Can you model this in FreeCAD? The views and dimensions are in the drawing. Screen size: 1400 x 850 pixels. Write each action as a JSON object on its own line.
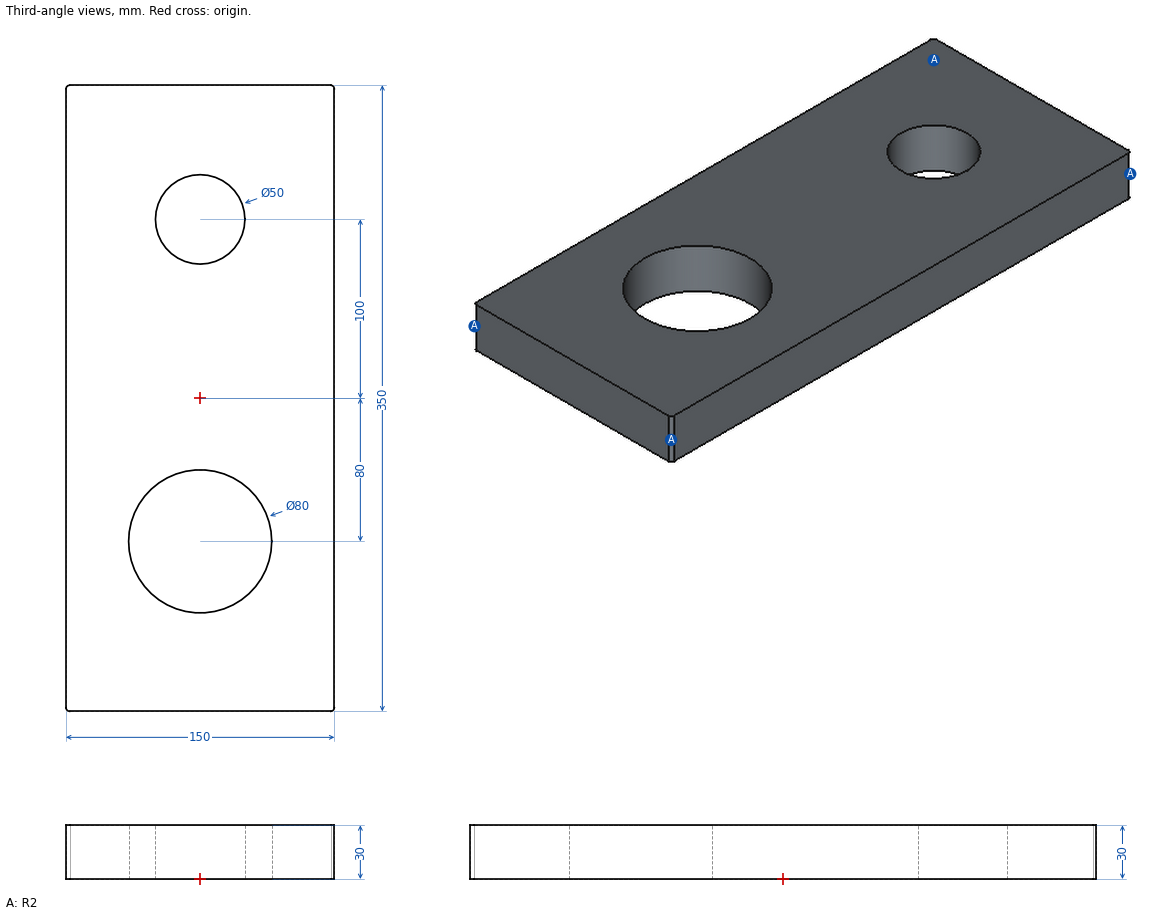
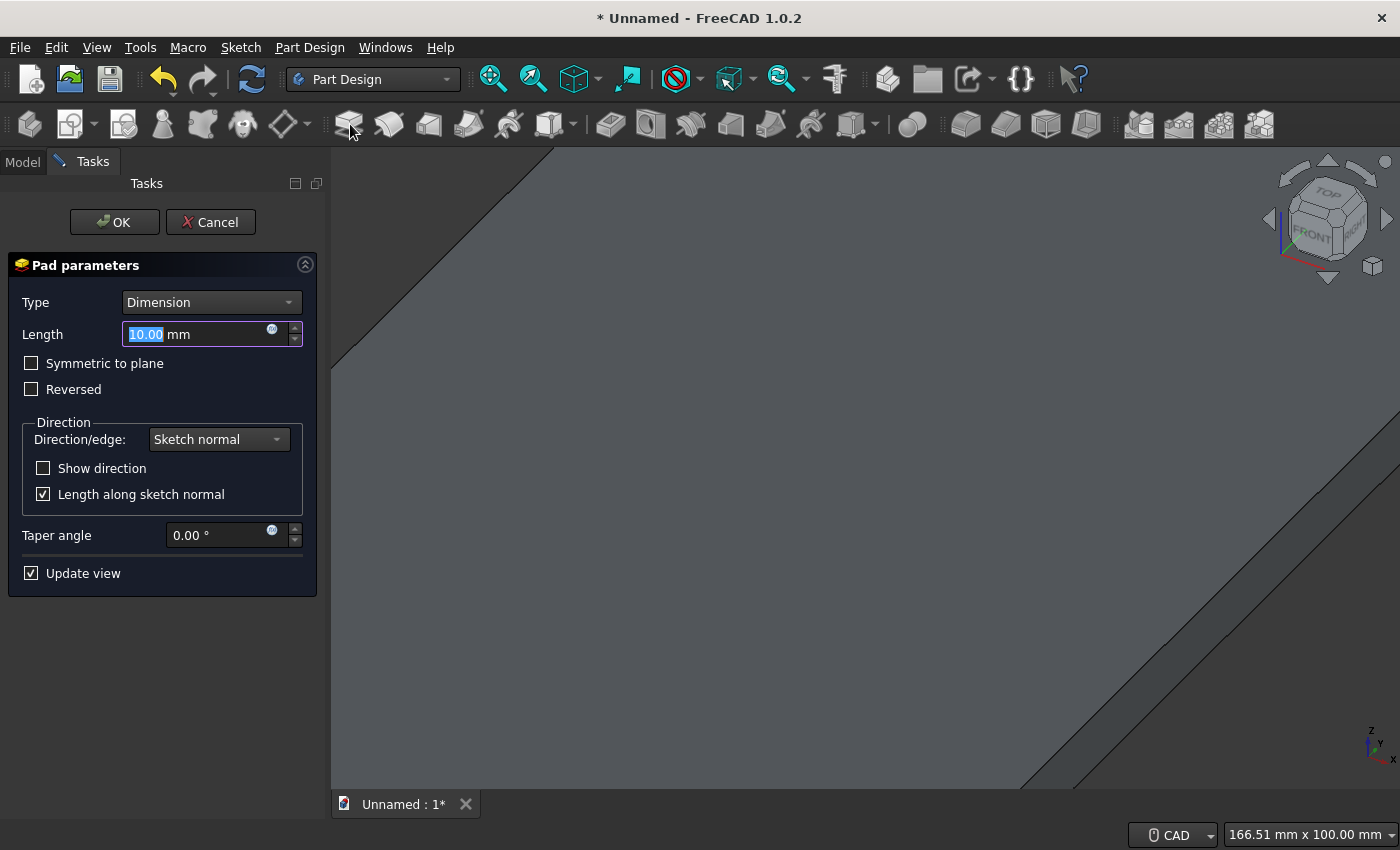
{"action": "type", "text": "30"}
{"action": "key", "text": "Tab"}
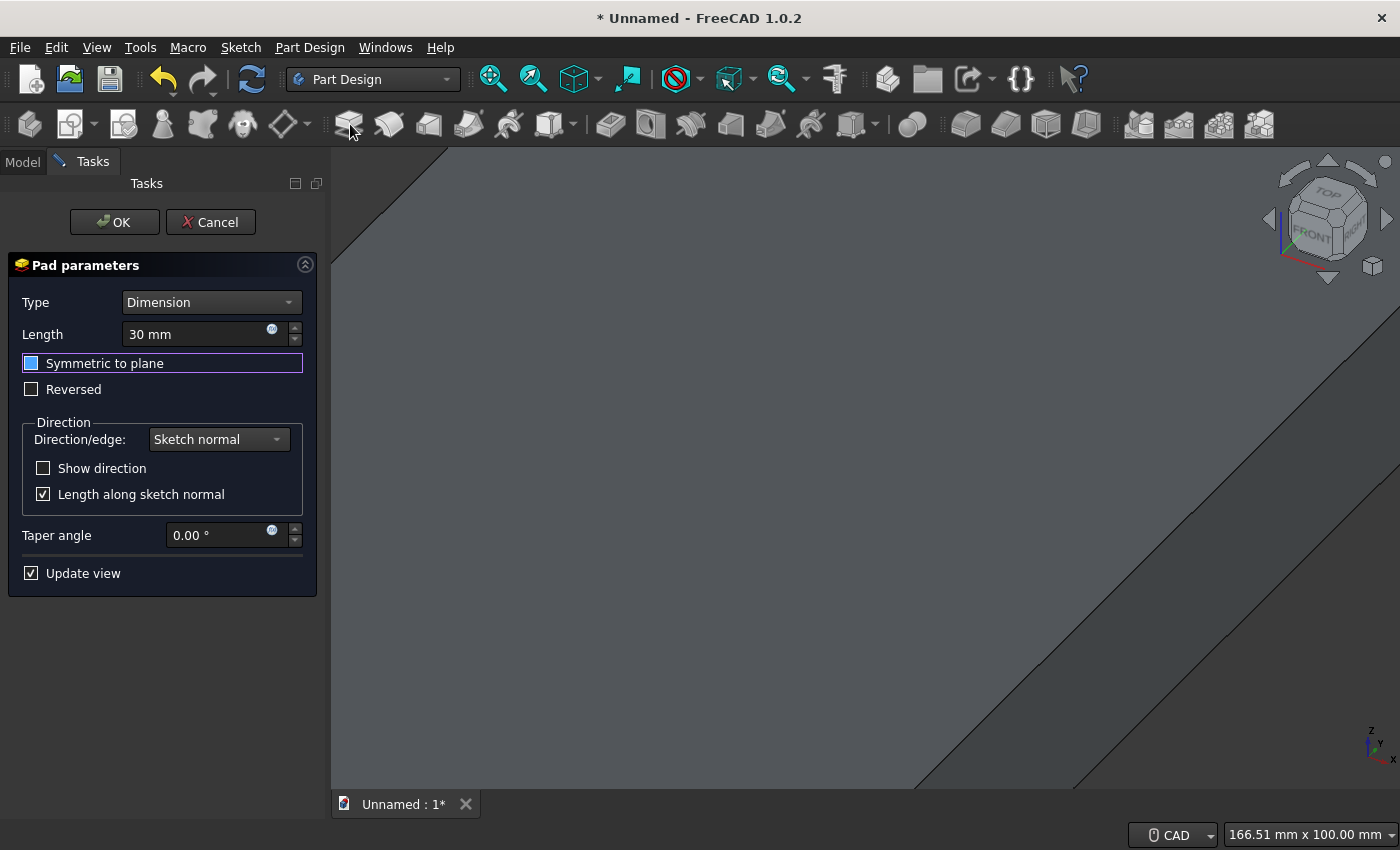
{"action": "left_click", "coordinate": [115, 222]}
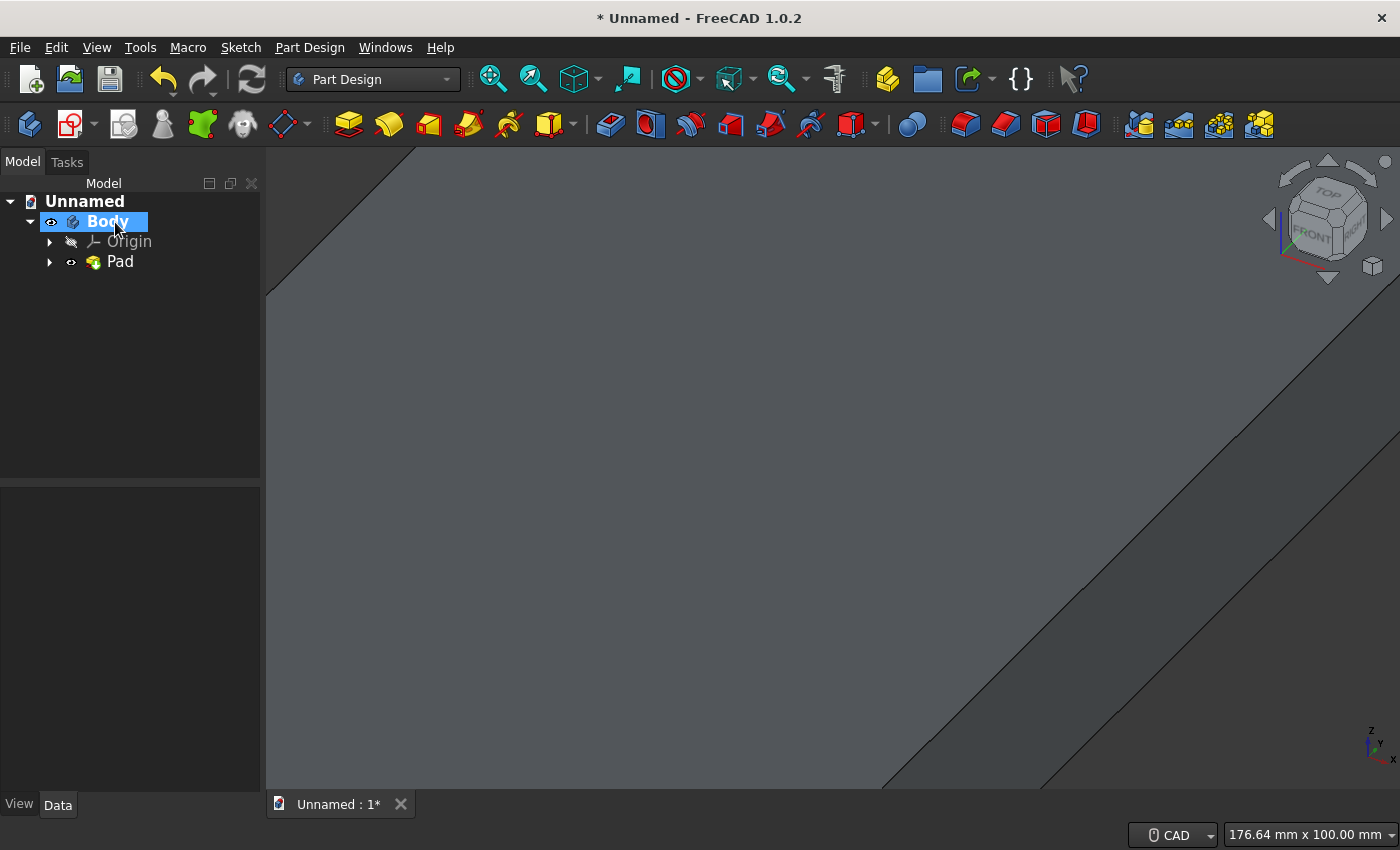
{"action": "left_click", "coordinate": [494, 80]}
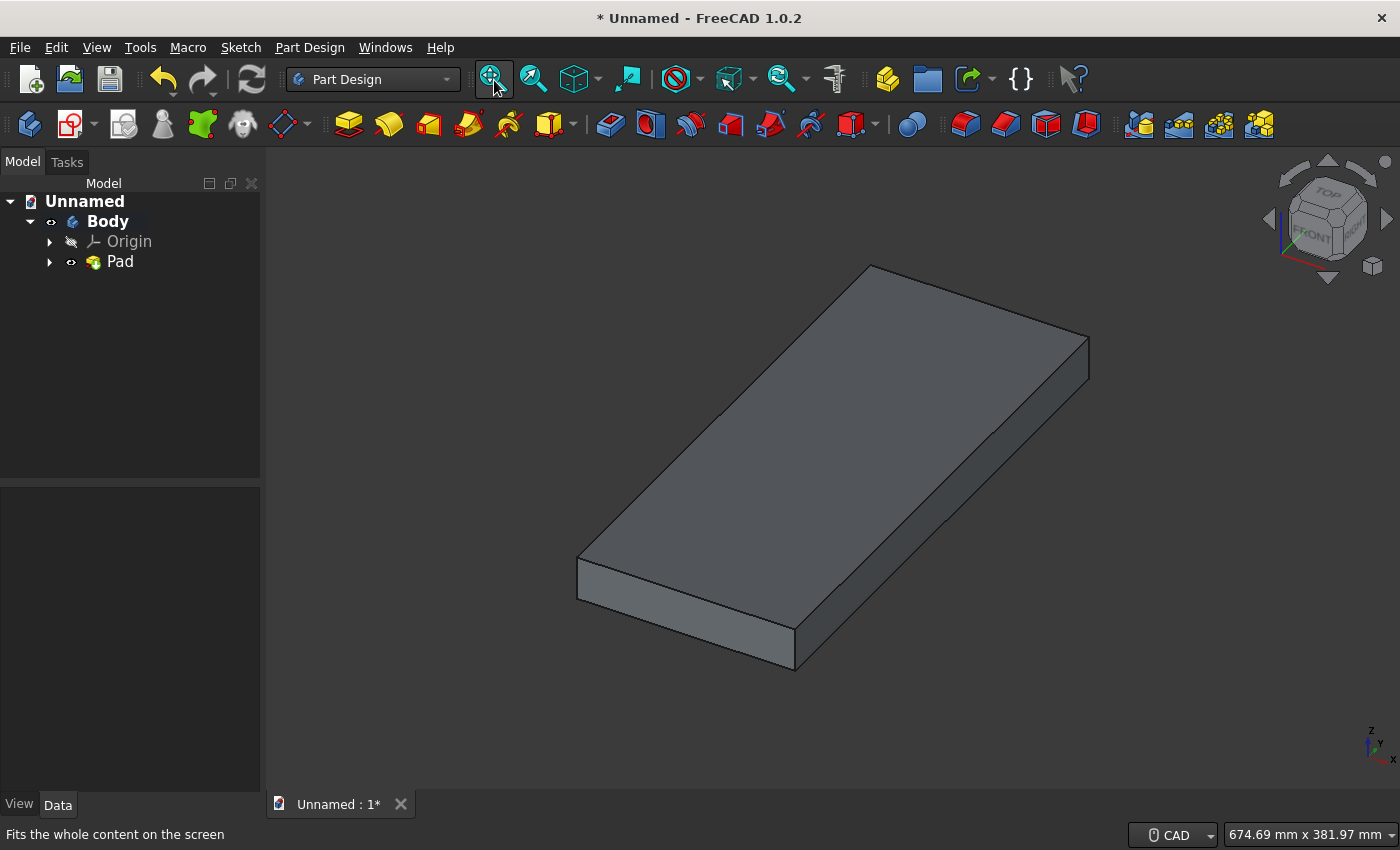
{"action": "left_click", "coordinate": [917, 363]}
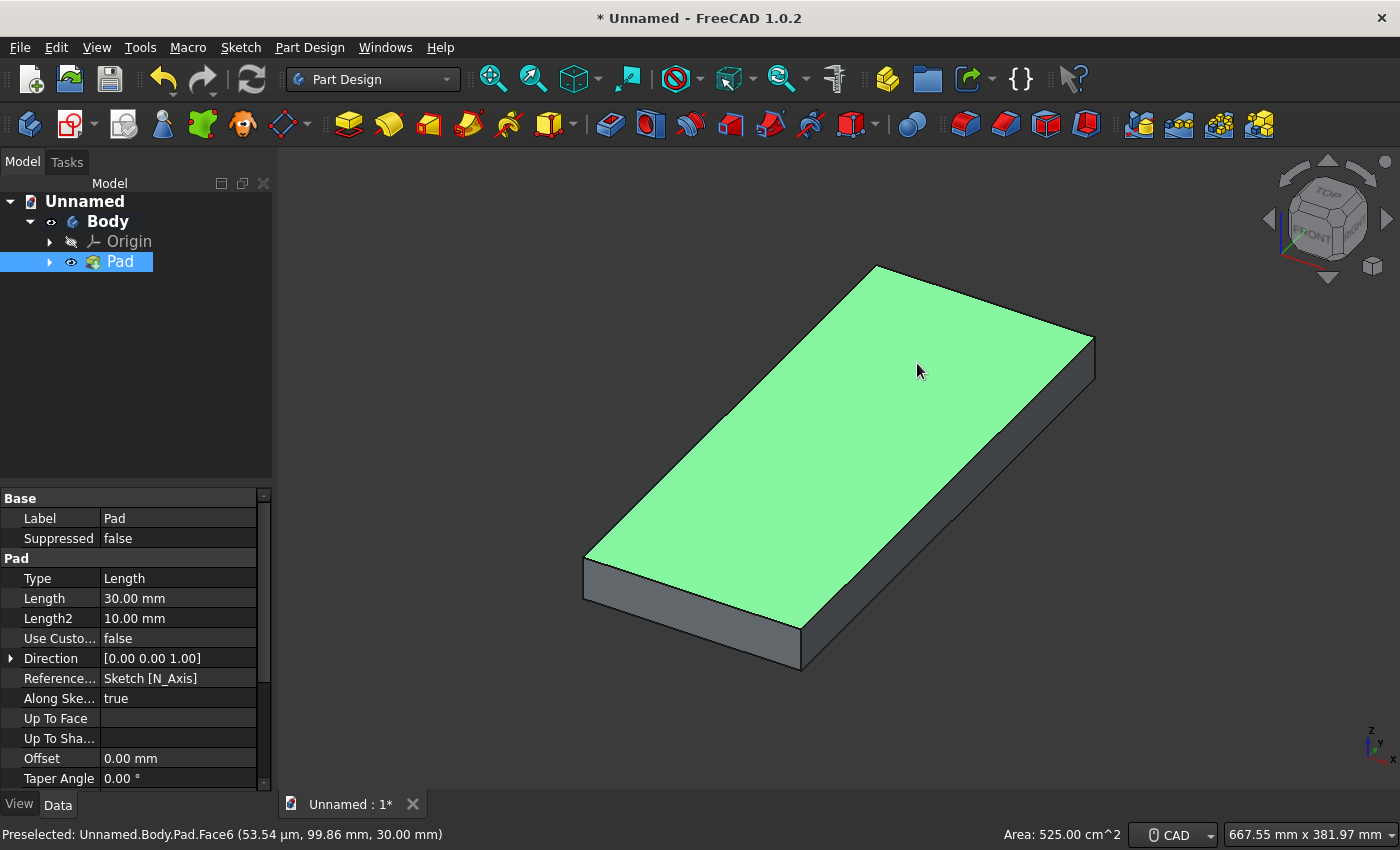
{"action": "left_click", "coordinate": [70, 124]}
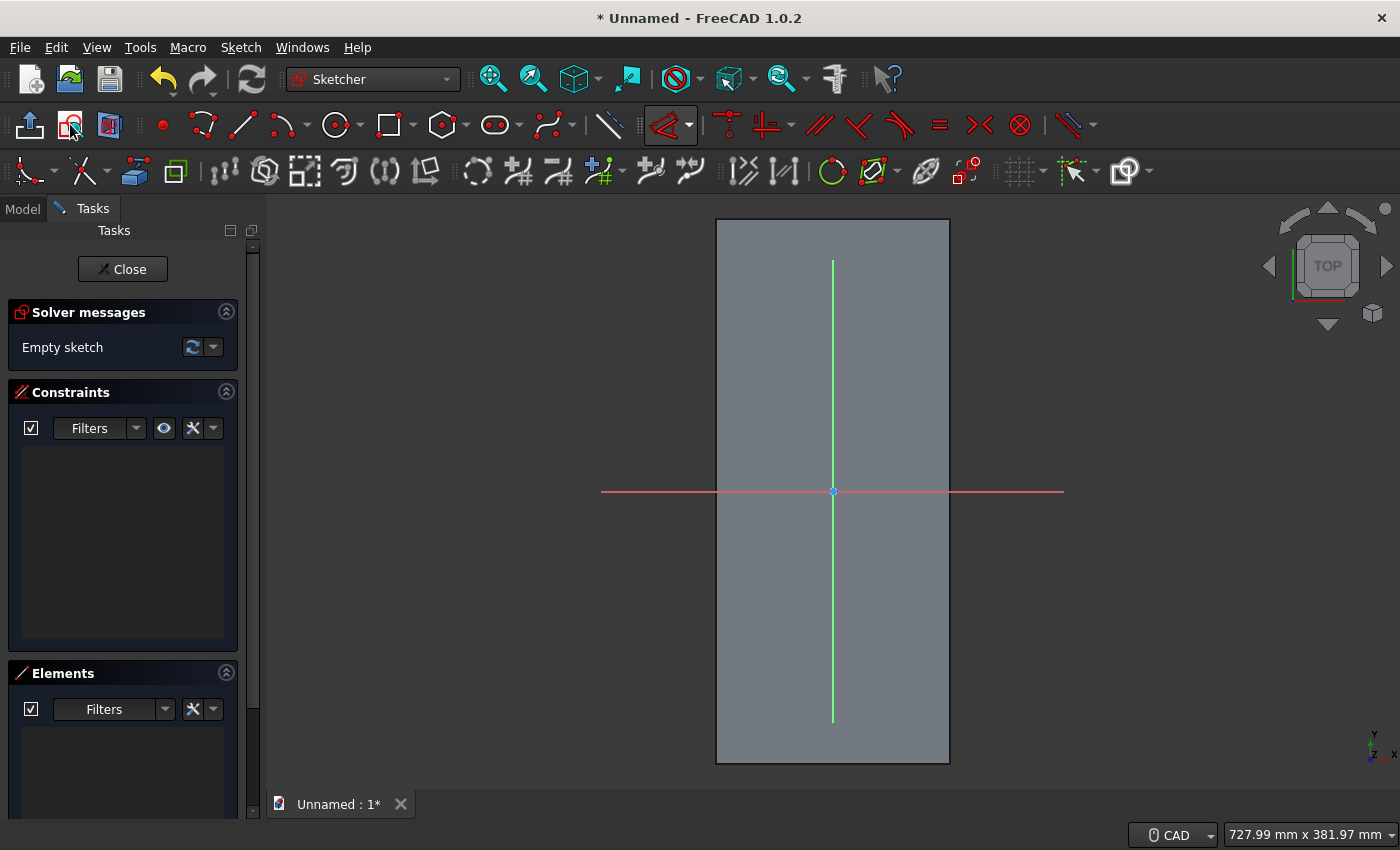
{"action": "left_click", "coordinate": [336, 126]}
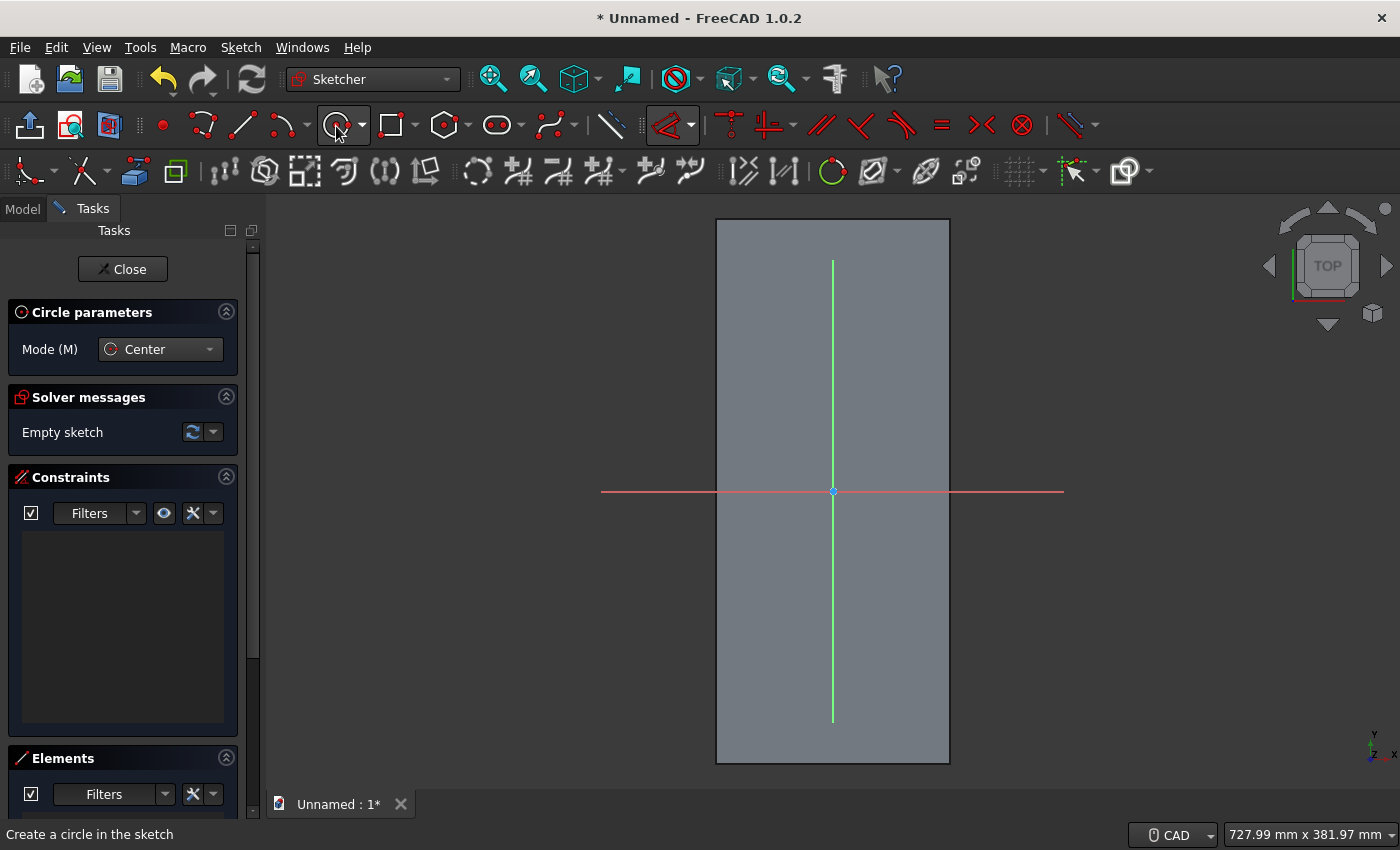
{"action": "left_click", "coordinate": [833, 336]}
{"action": "left_click", "coordinate": [861, 308]}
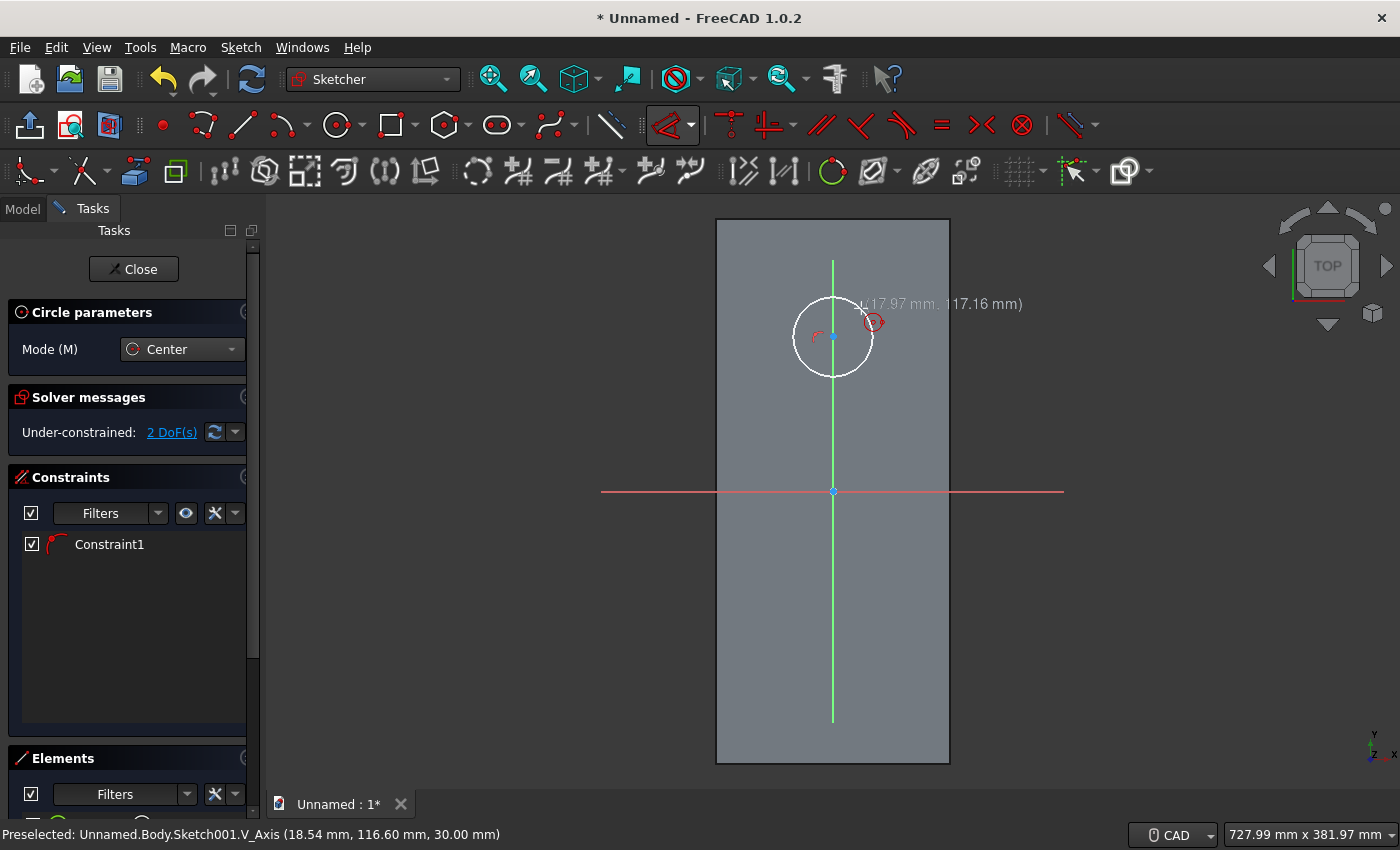
{"action": "left_click", "coordinate": [833, 616]}
{"action": "left_click", "coordinate": [877, 572]}
{"action": "key", "text": "Escape"}